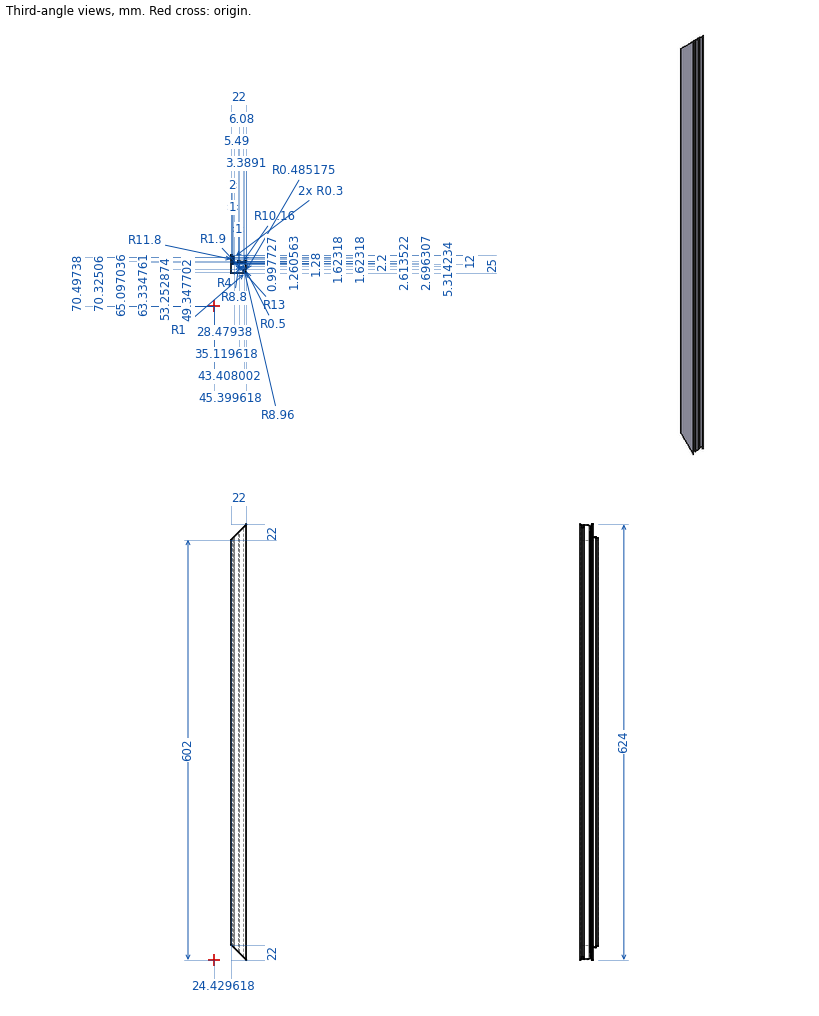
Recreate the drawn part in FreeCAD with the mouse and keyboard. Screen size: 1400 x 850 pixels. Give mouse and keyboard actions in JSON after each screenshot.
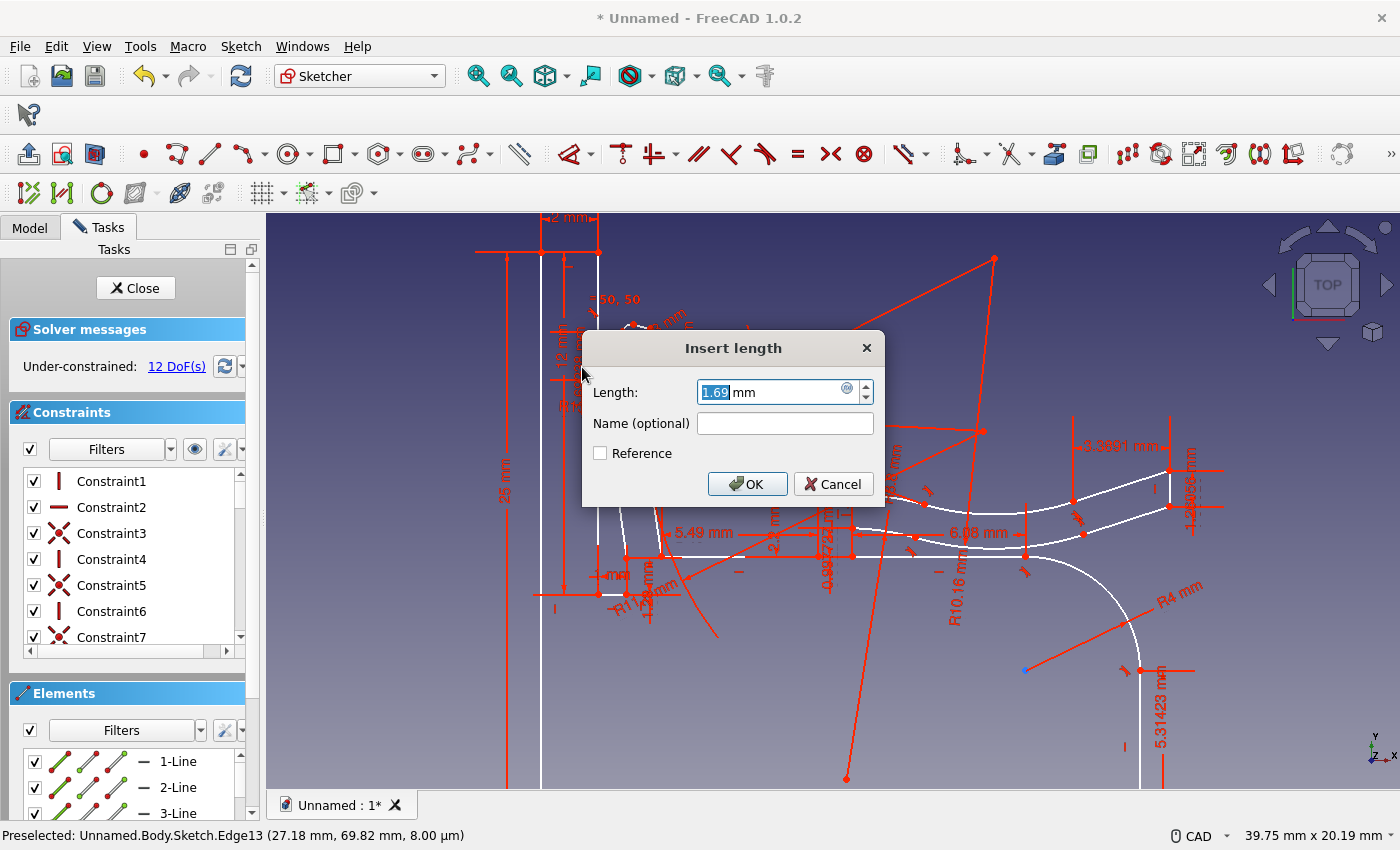
{"action": "type", "text": "1.62318"}
{"action": "key", "text": "Return"}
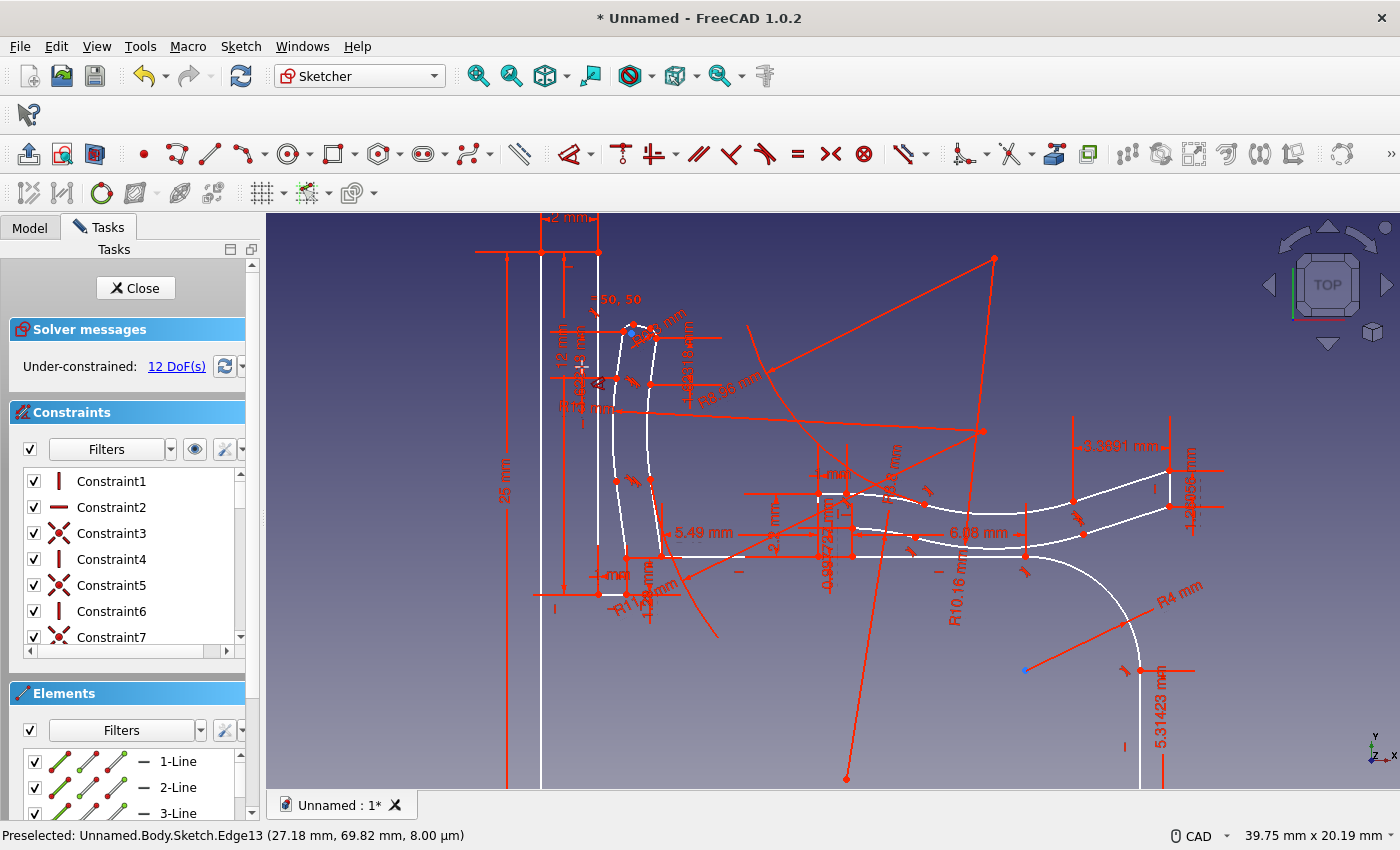
{"action": "scroll", "coordinate": [657, 338], "scroll_direction": "up", "scroll_amount": 2}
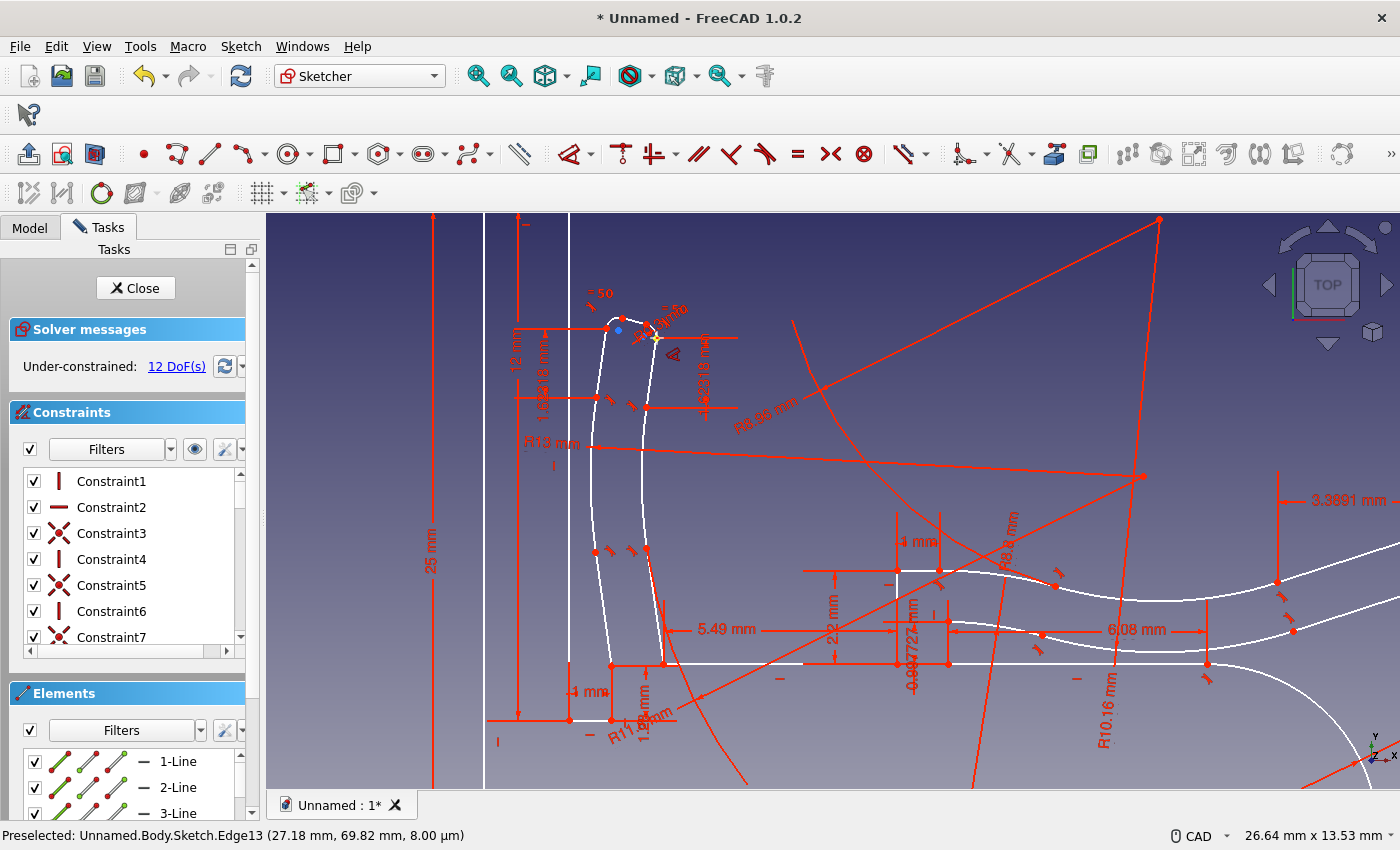
{"action": "left_click", "coordinate": [656, 338]}
{"action": "left_click", "coordinate": [392, 304]}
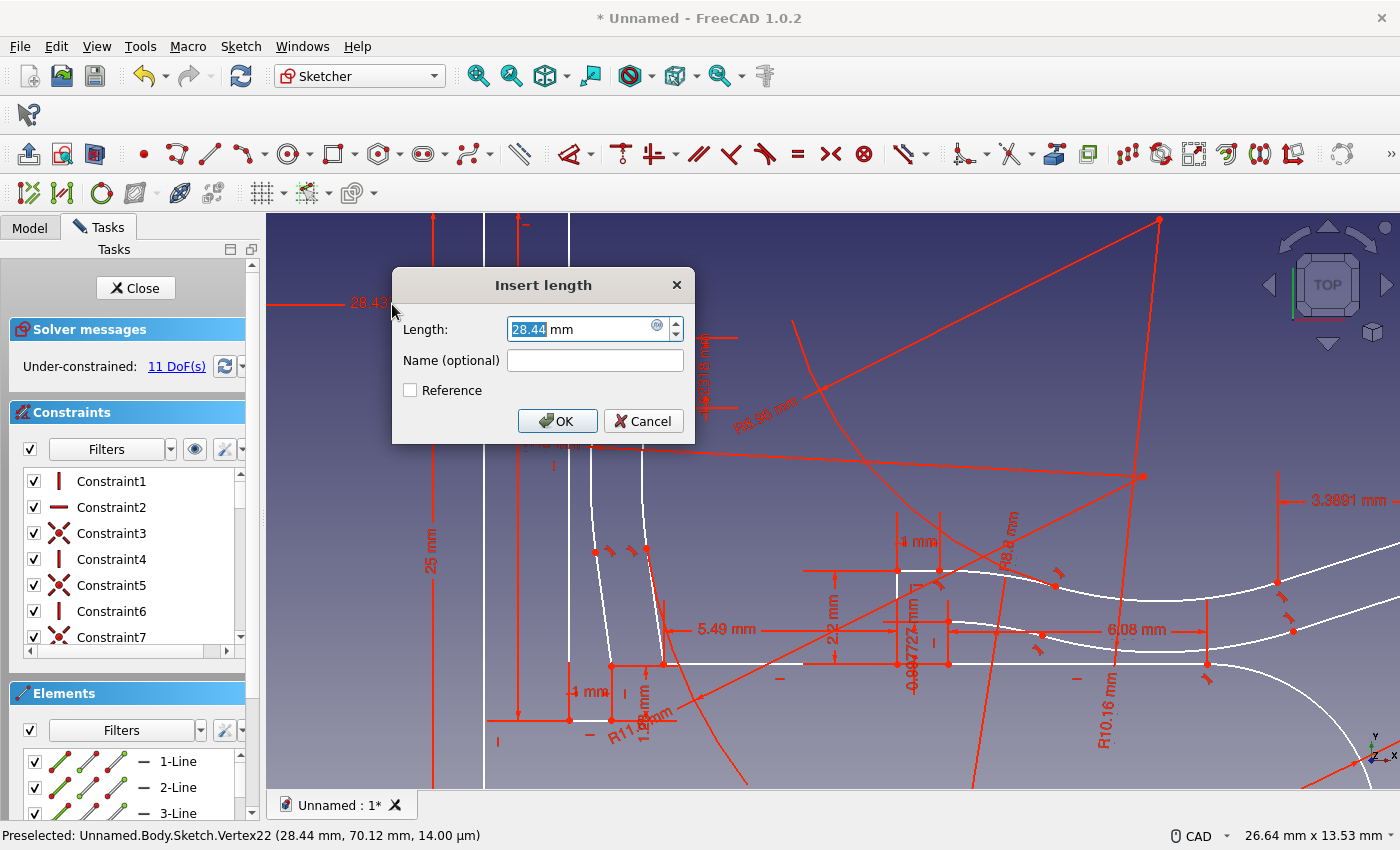
{"action": "type", "text": "28.47938"}
{"action": "key", "text": "Return"}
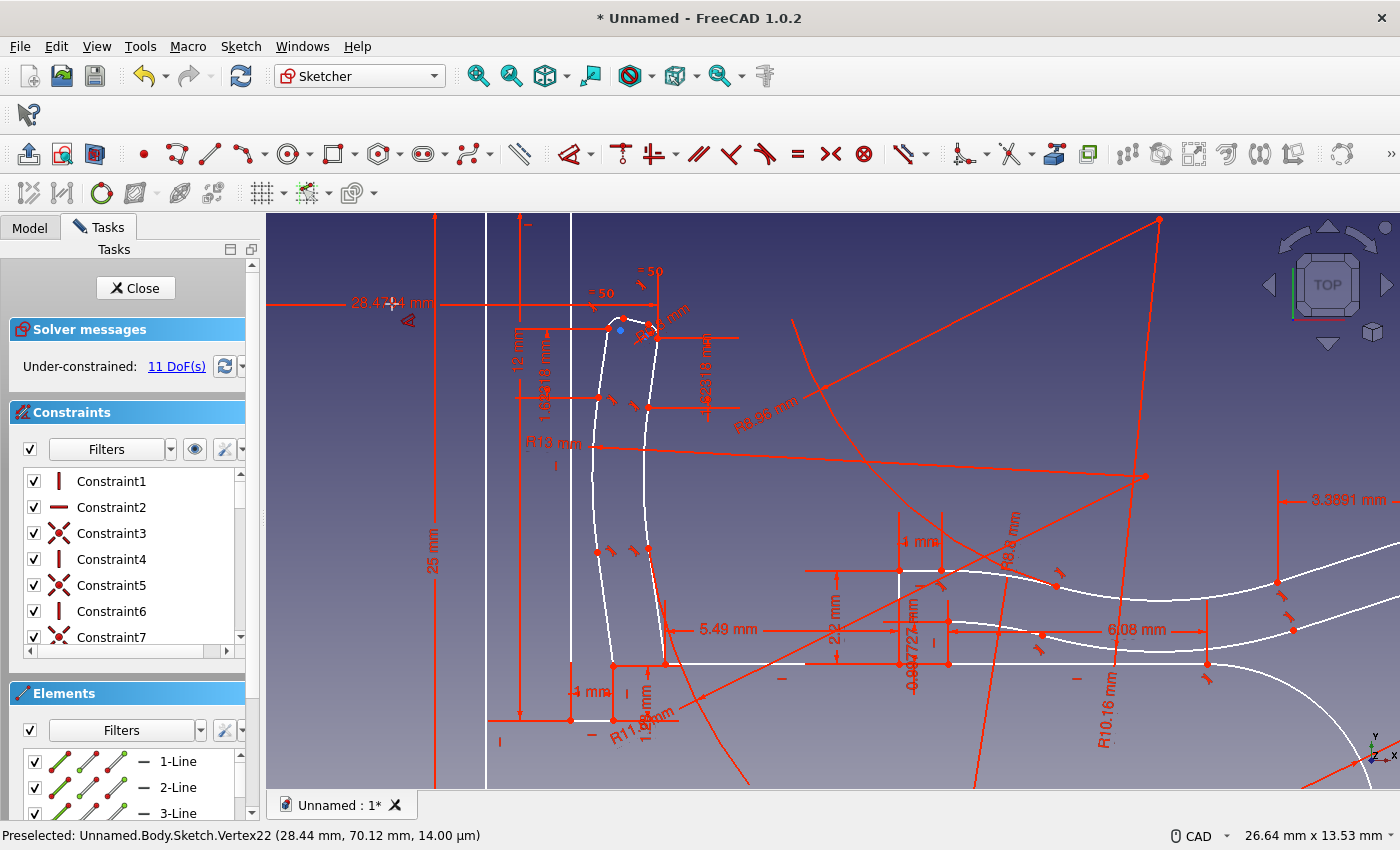
{"action": "left_click", "coordinate": [648, 324]}
{"action": "left_click", "coordinate": [682, 543]}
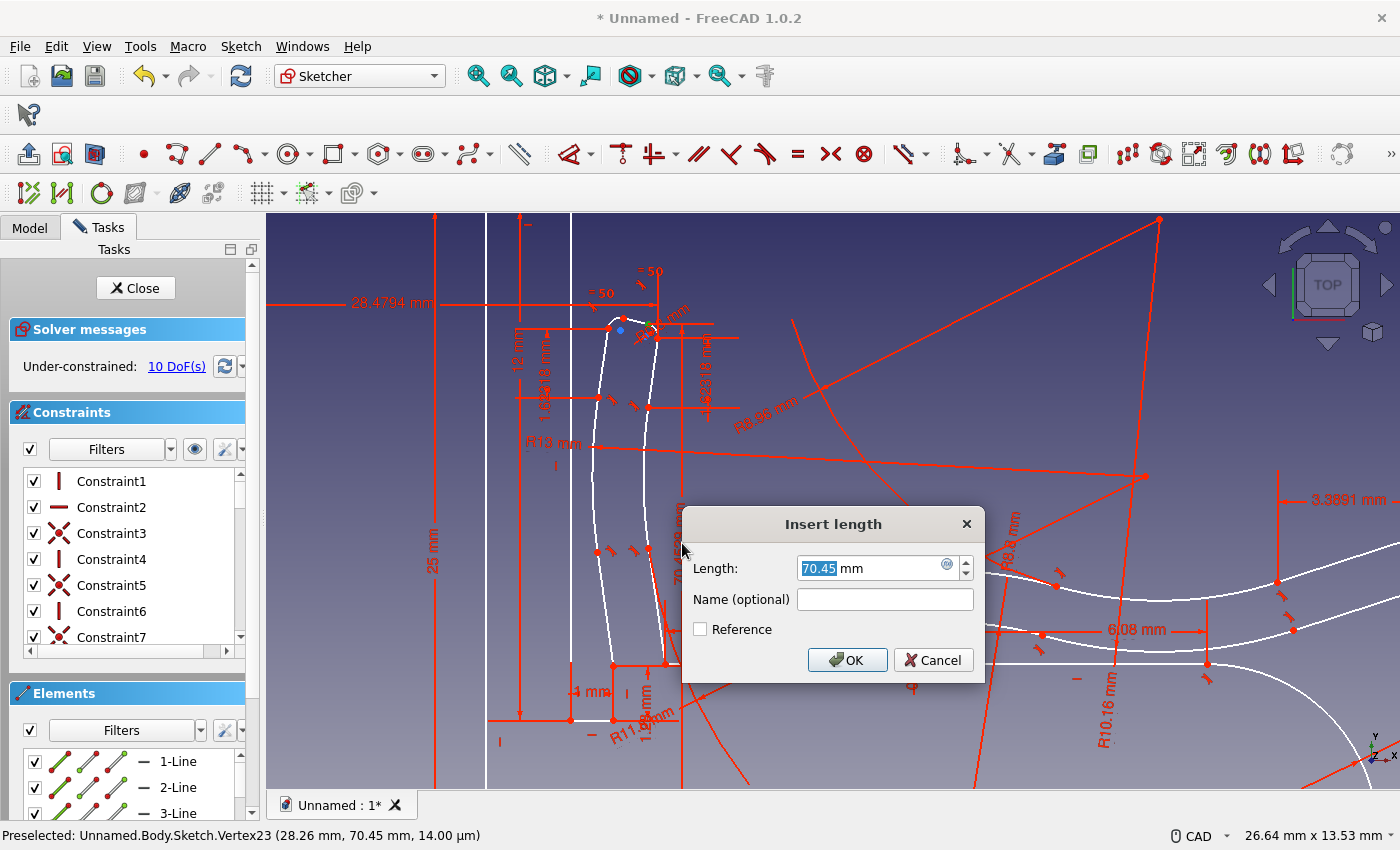
{"action": "type", "text": "70.49738"}
{"action": "key", "text": "Return"}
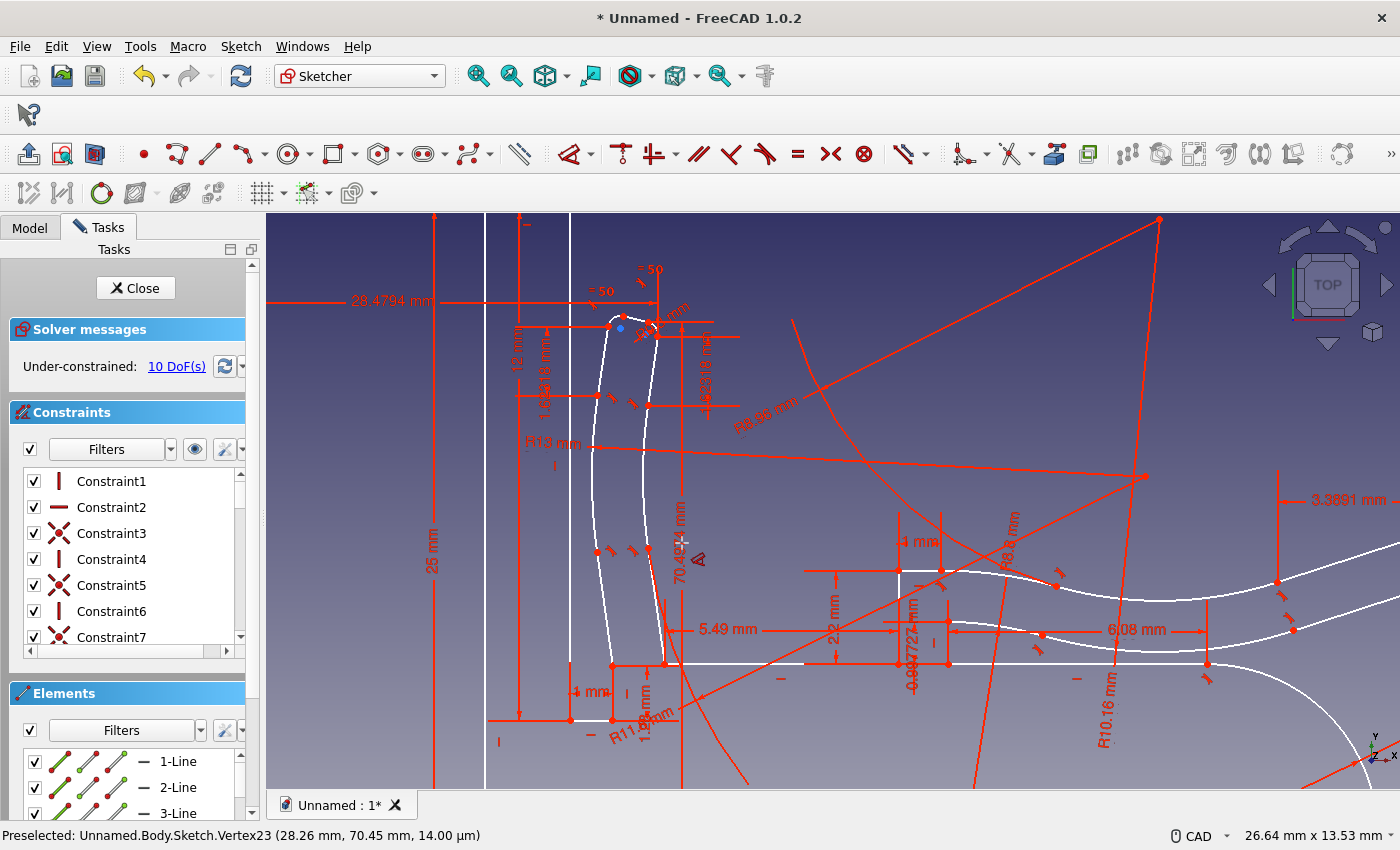
{"action": "left_click", "coordinate": [608, 327]}
{"action": "left_click", "coordinate": [642, 644]}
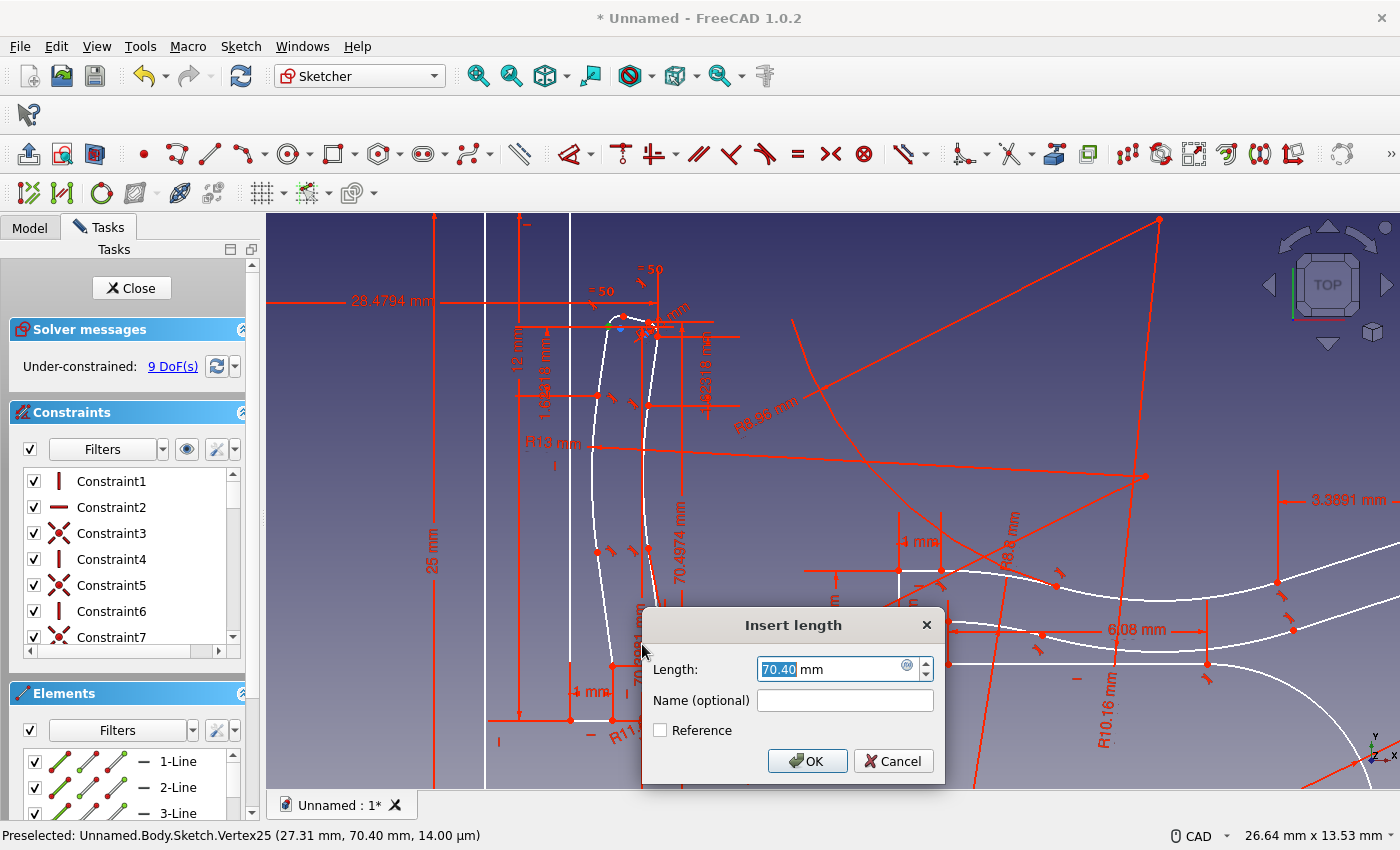
{"action": "type", "text": "70.32506"}
{"action": "key", "text": "Return"}